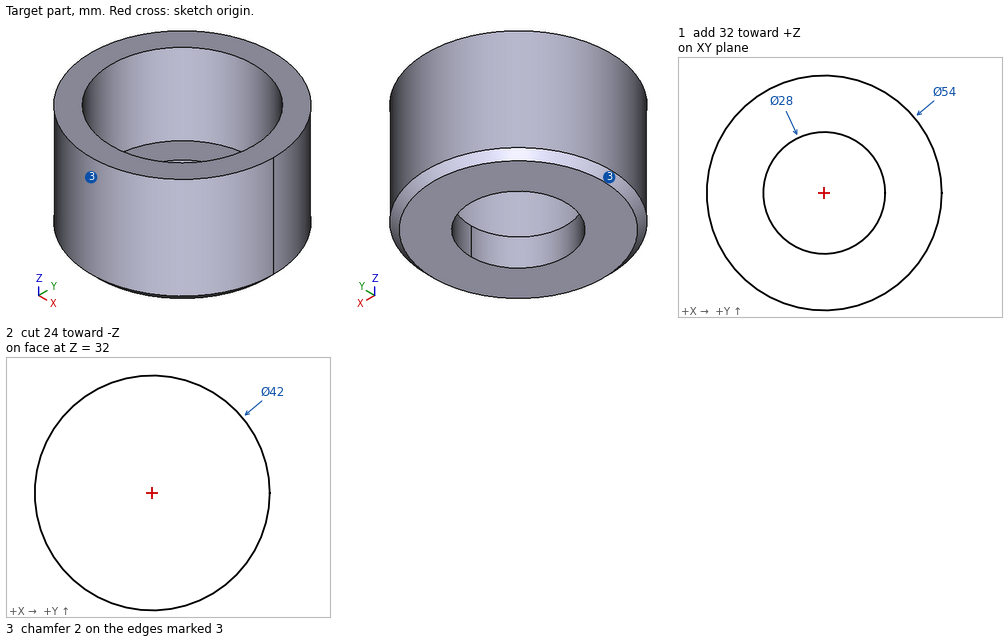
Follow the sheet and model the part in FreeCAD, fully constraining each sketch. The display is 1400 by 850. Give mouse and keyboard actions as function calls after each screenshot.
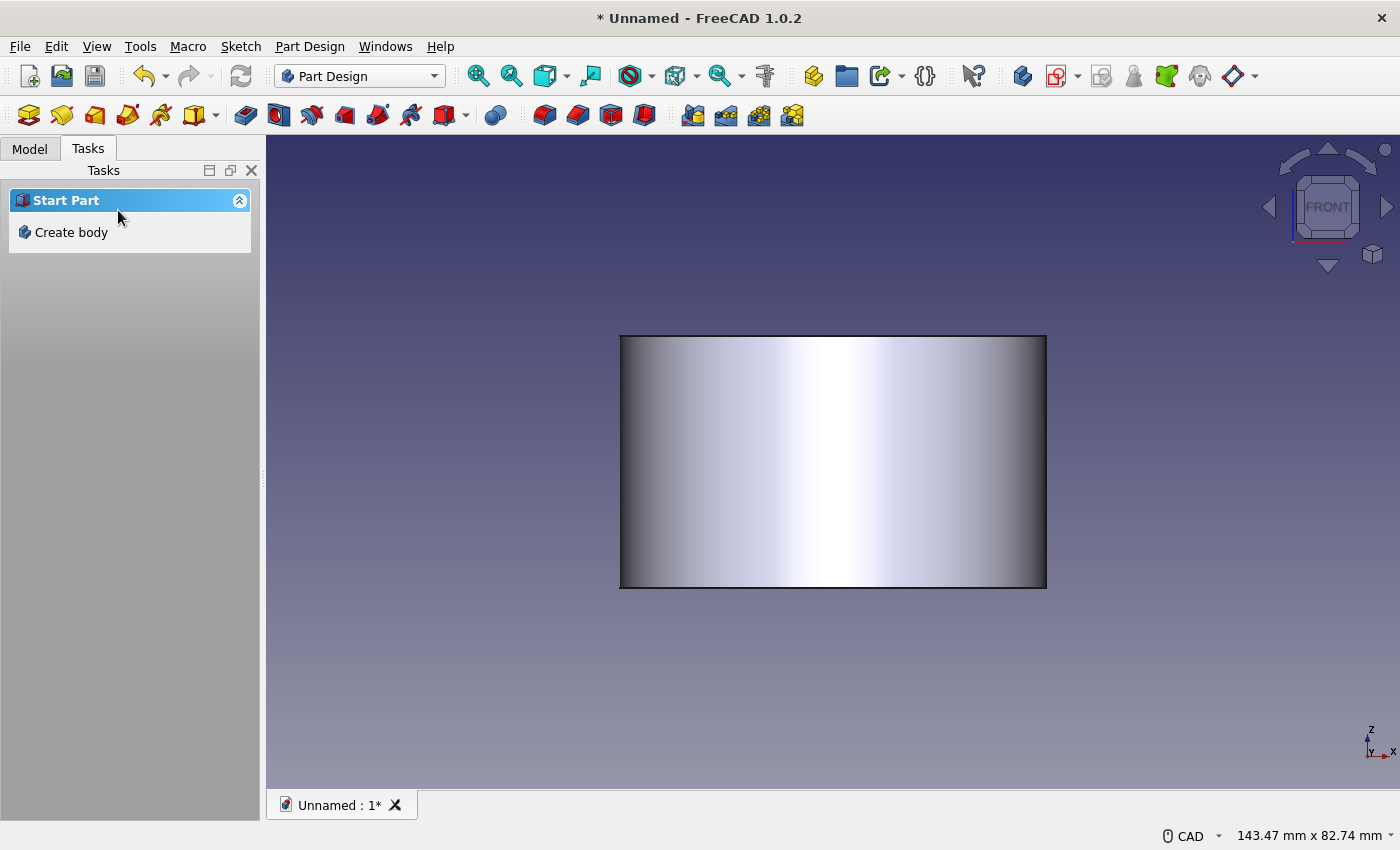
click(660, 587)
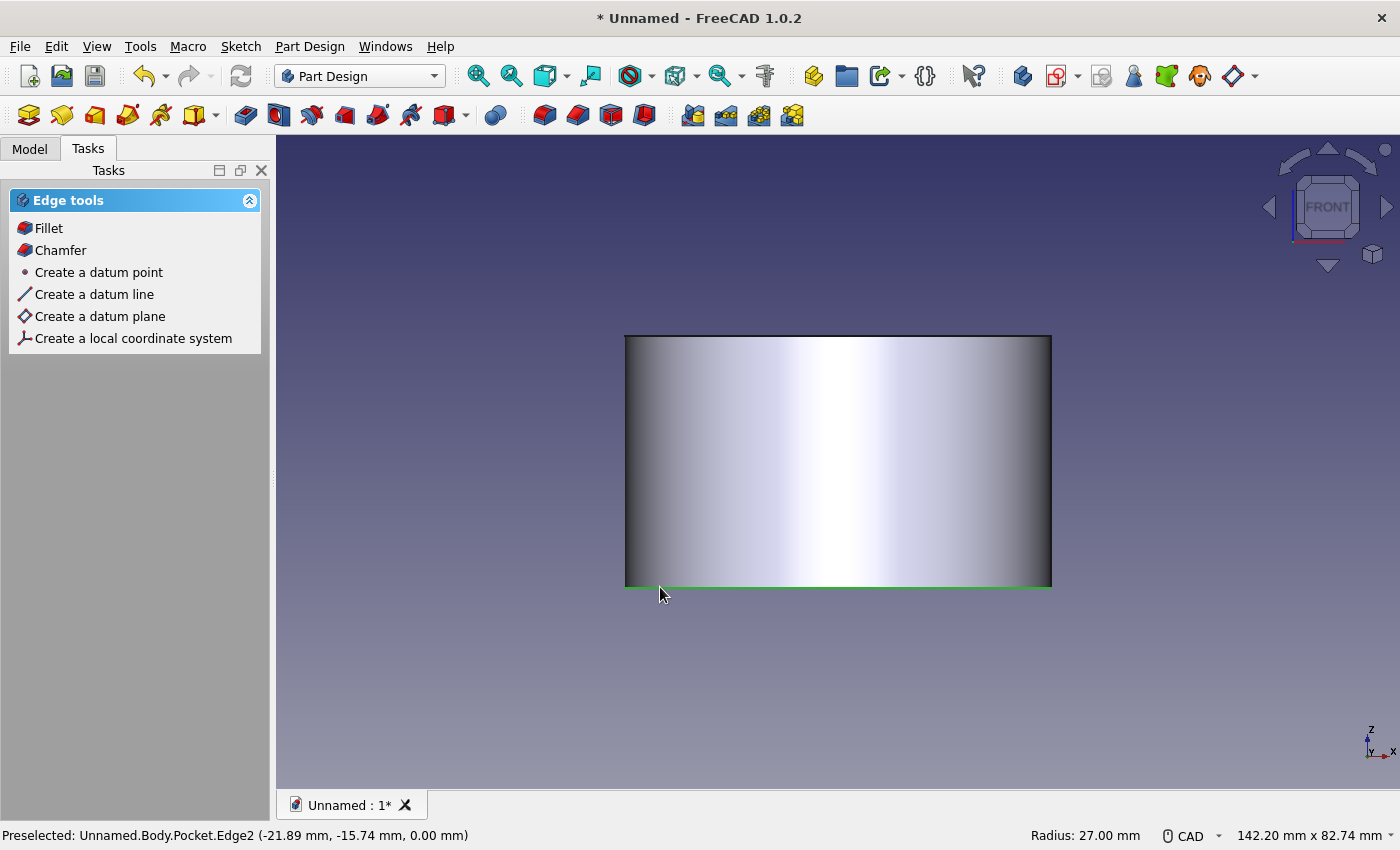
click(578, 116)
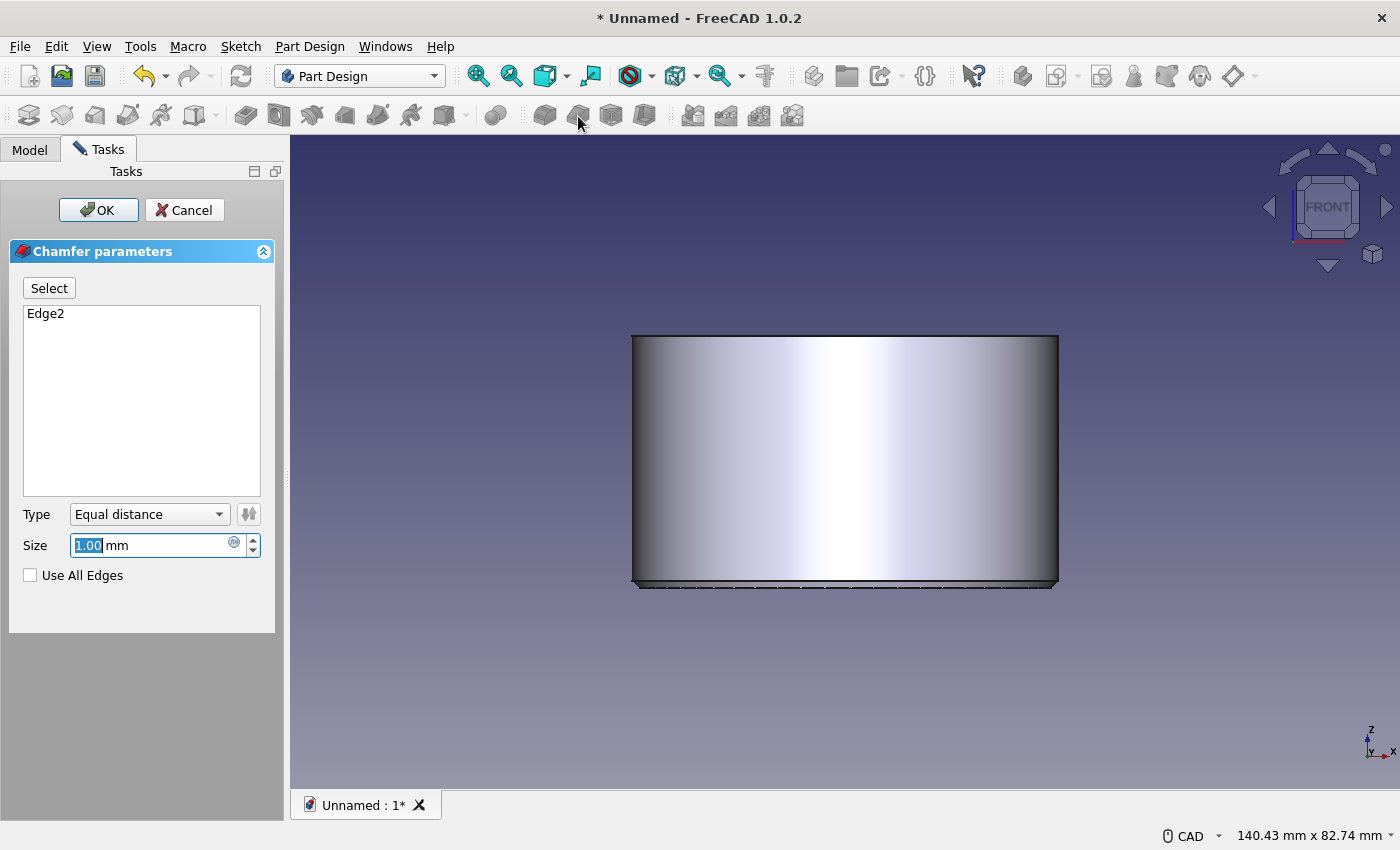
text(2)
key(Tab)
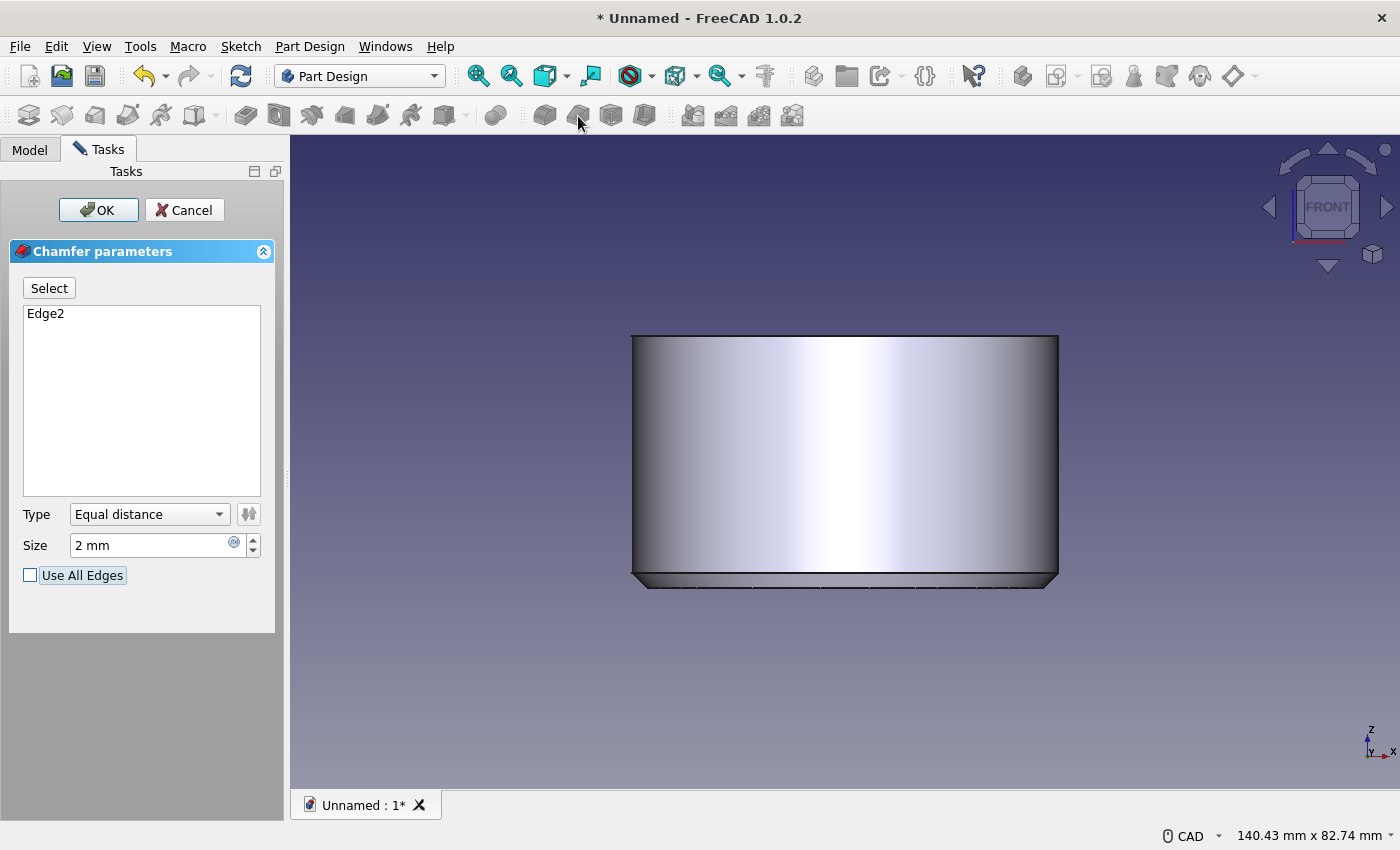
click(99, 210)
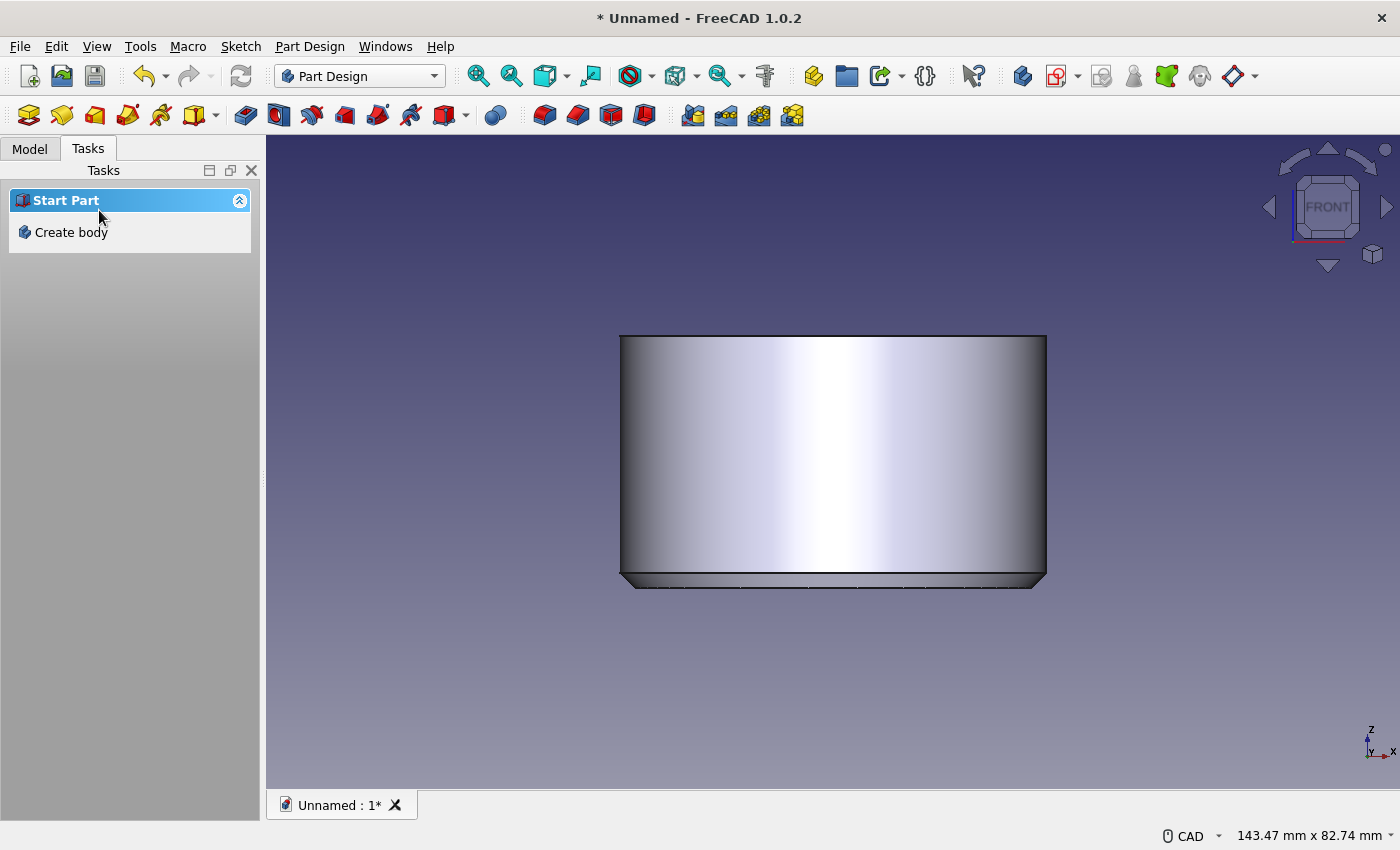
key(0)